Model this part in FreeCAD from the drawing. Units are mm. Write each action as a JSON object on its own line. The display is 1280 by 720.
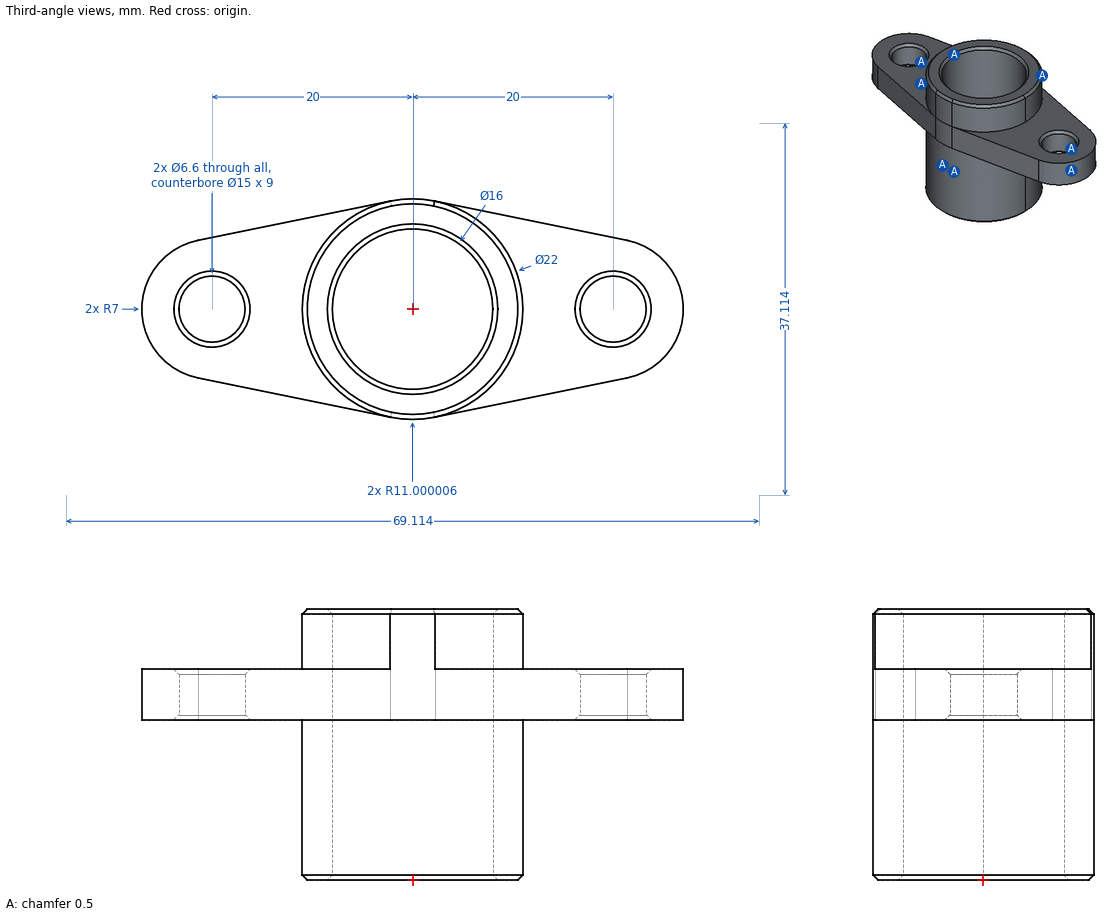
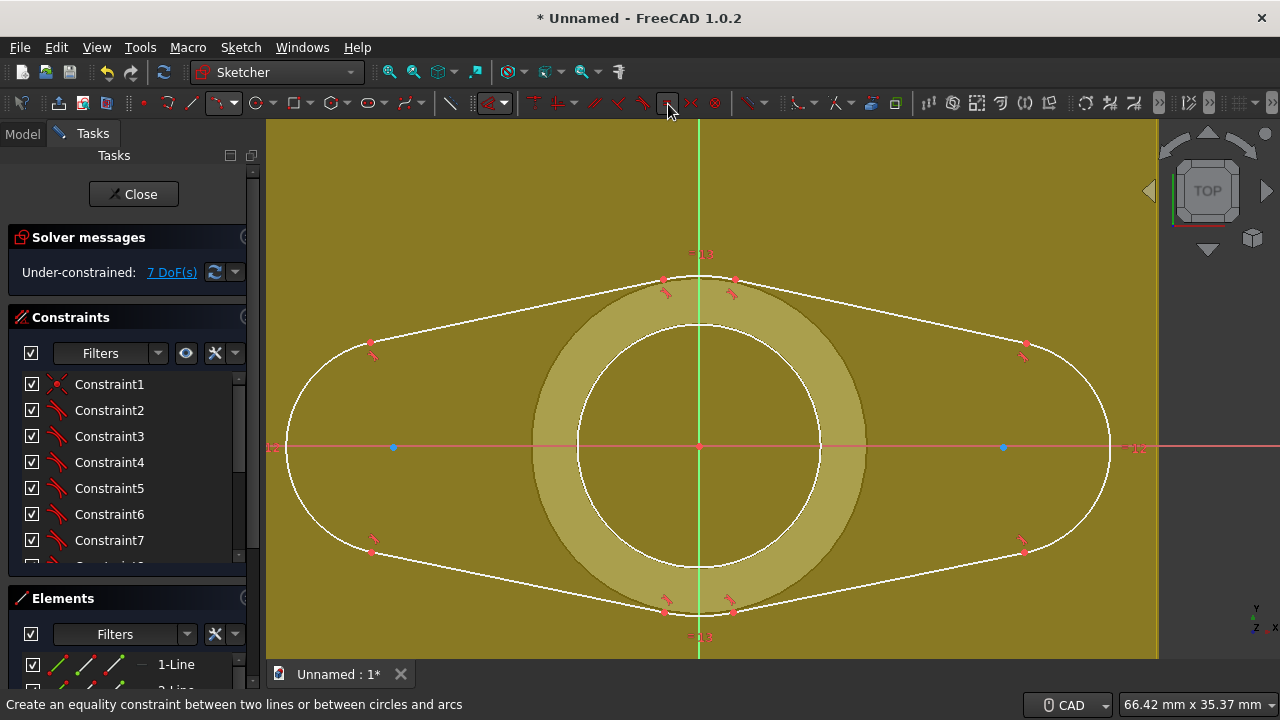
{"action": "left_click", "coordinate": [393, 447]}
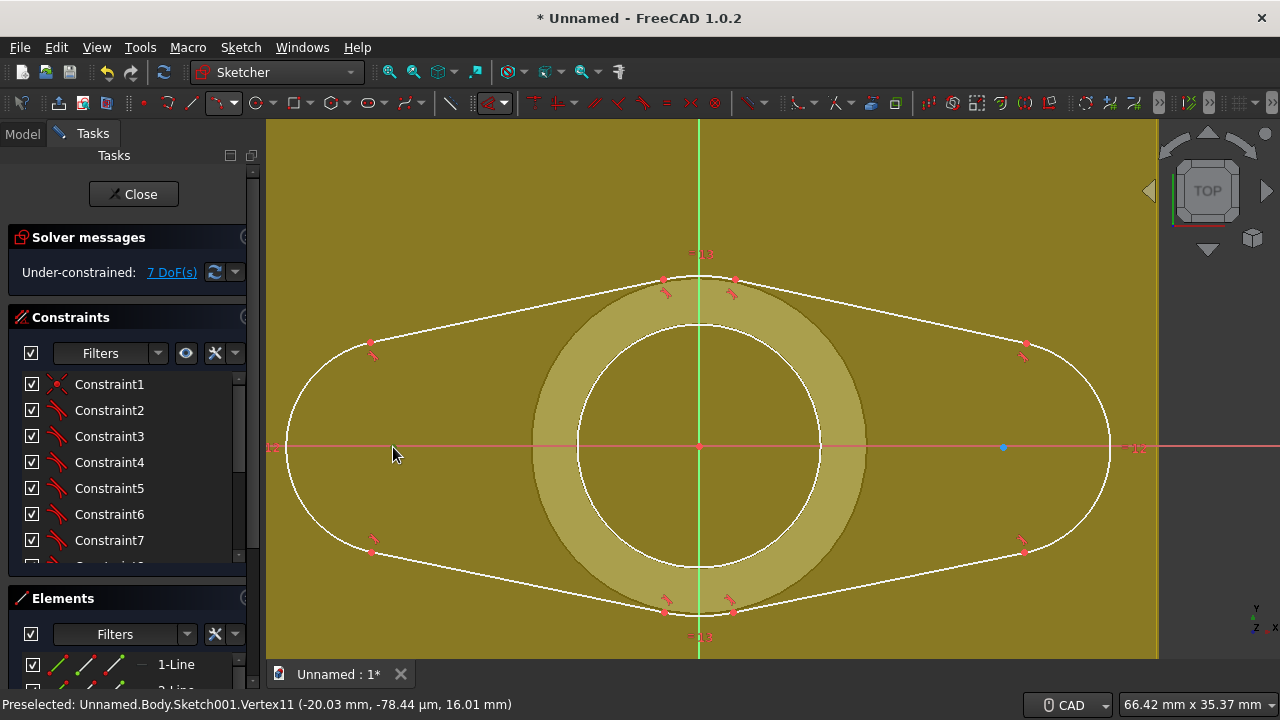
{"action": "left_click", "coordinate": [353, 446]}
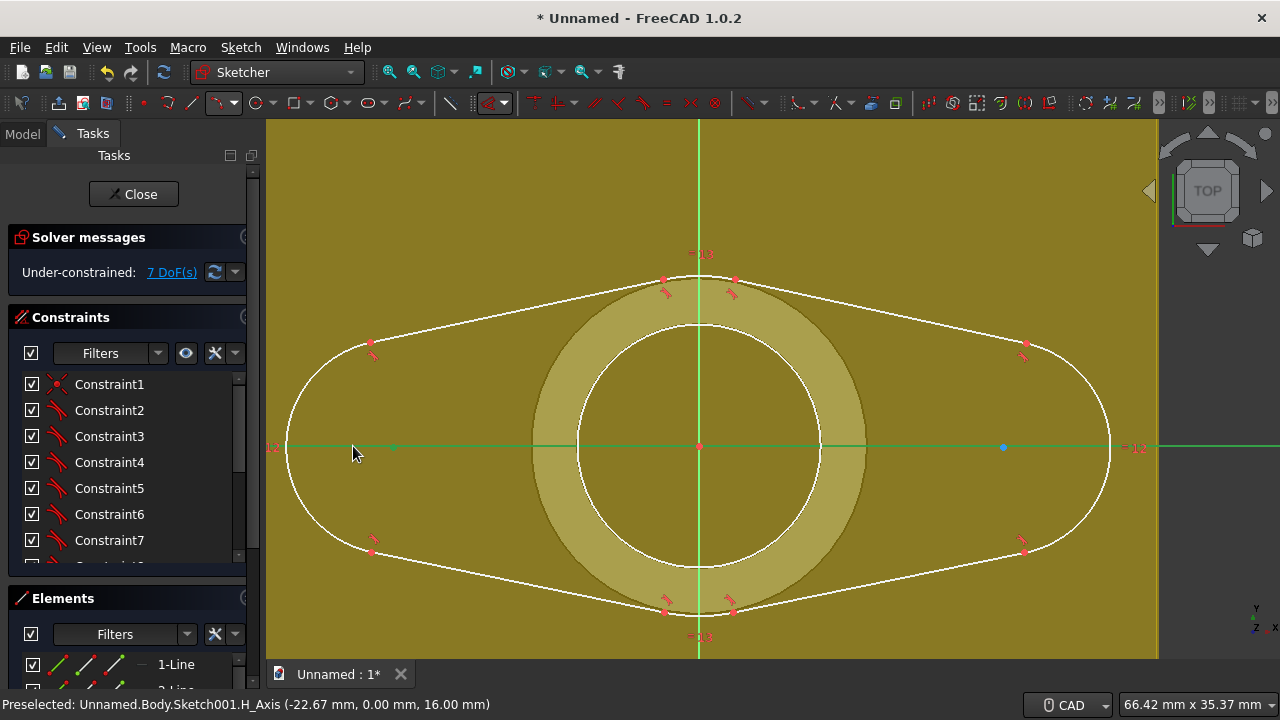
{"action": "left_click", "coordinate": [534, 104]}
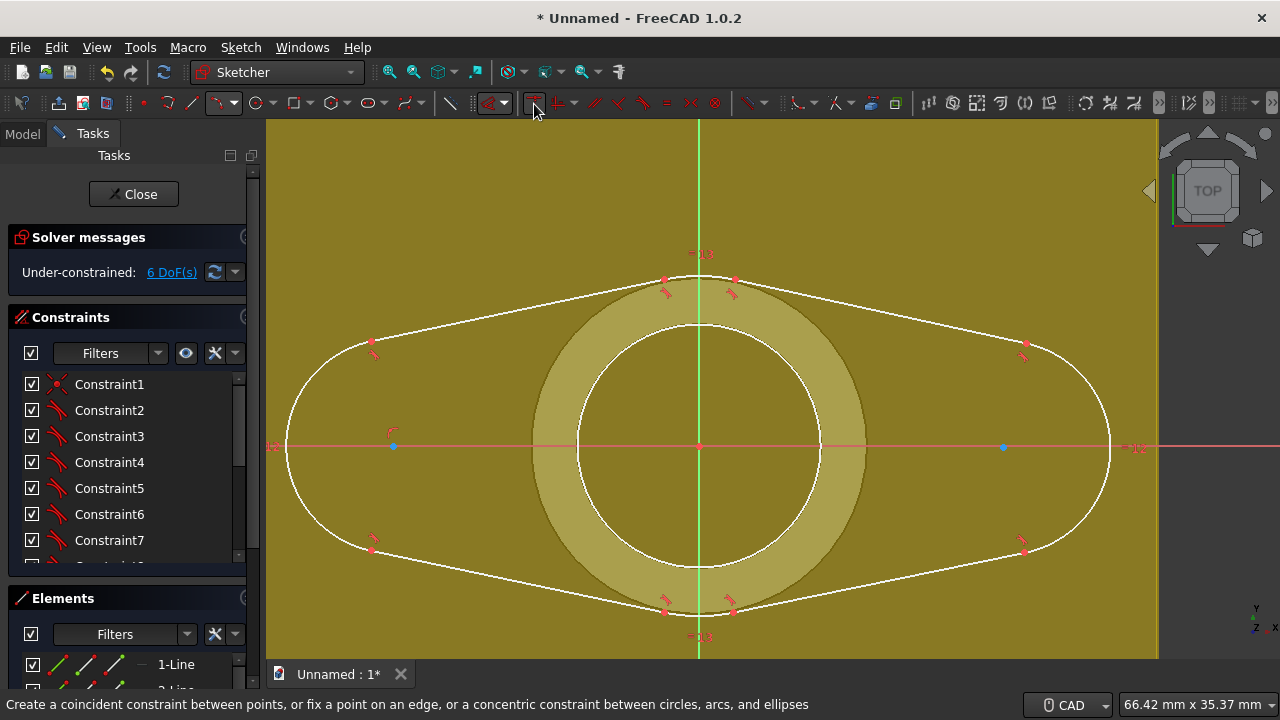
{"action": "left_click", "coordinate": [1003, 448]}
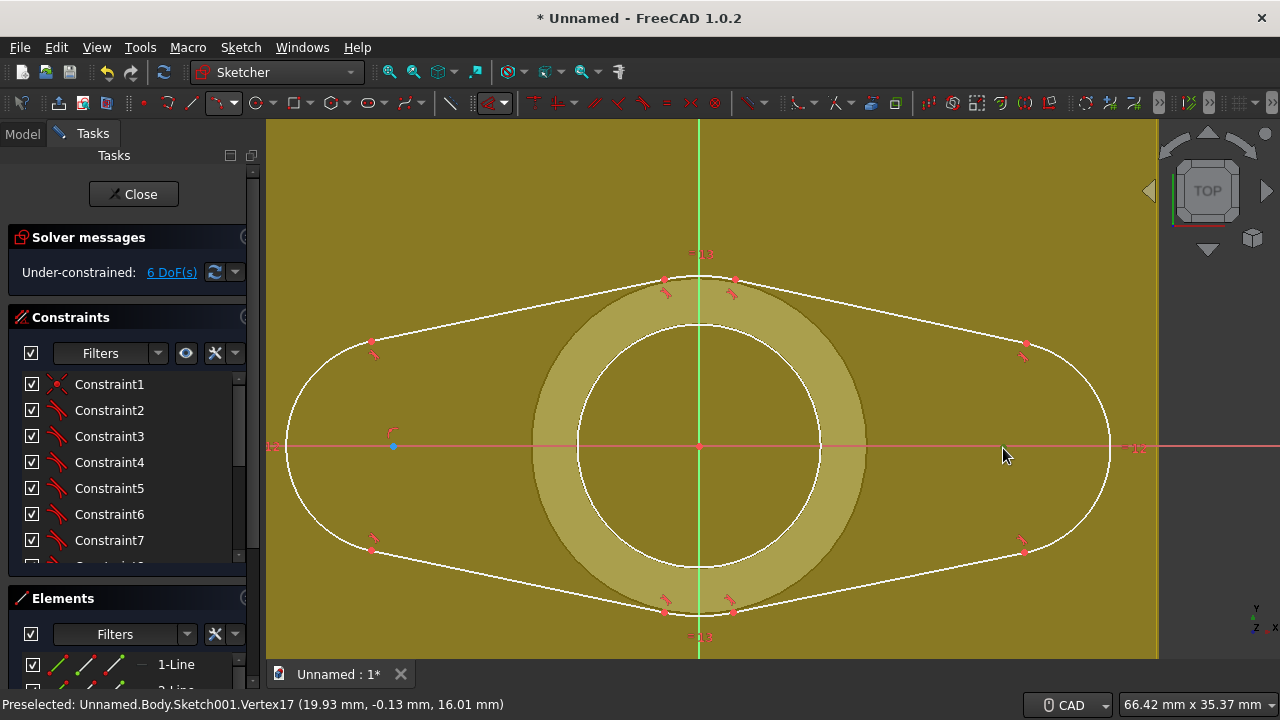
{"action": "left_click", "coordinate": [353, 446]}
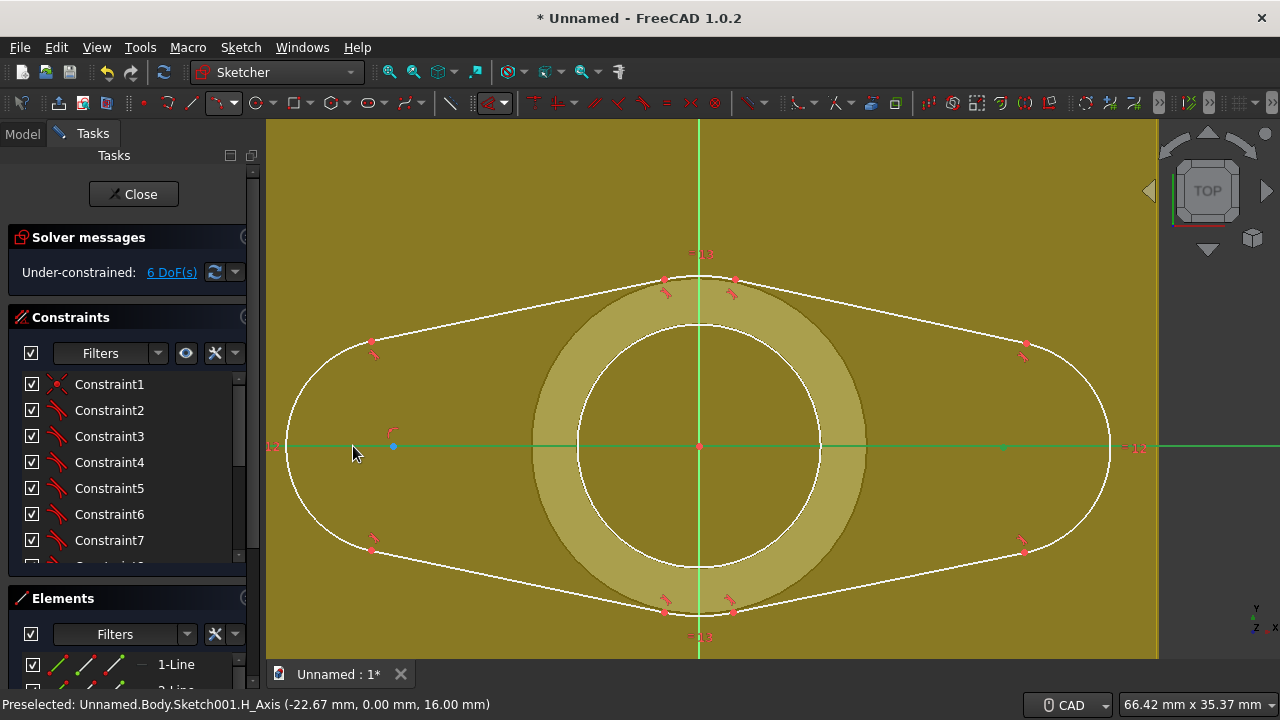
{"action": "left_click", "coordinate": [534, 104]}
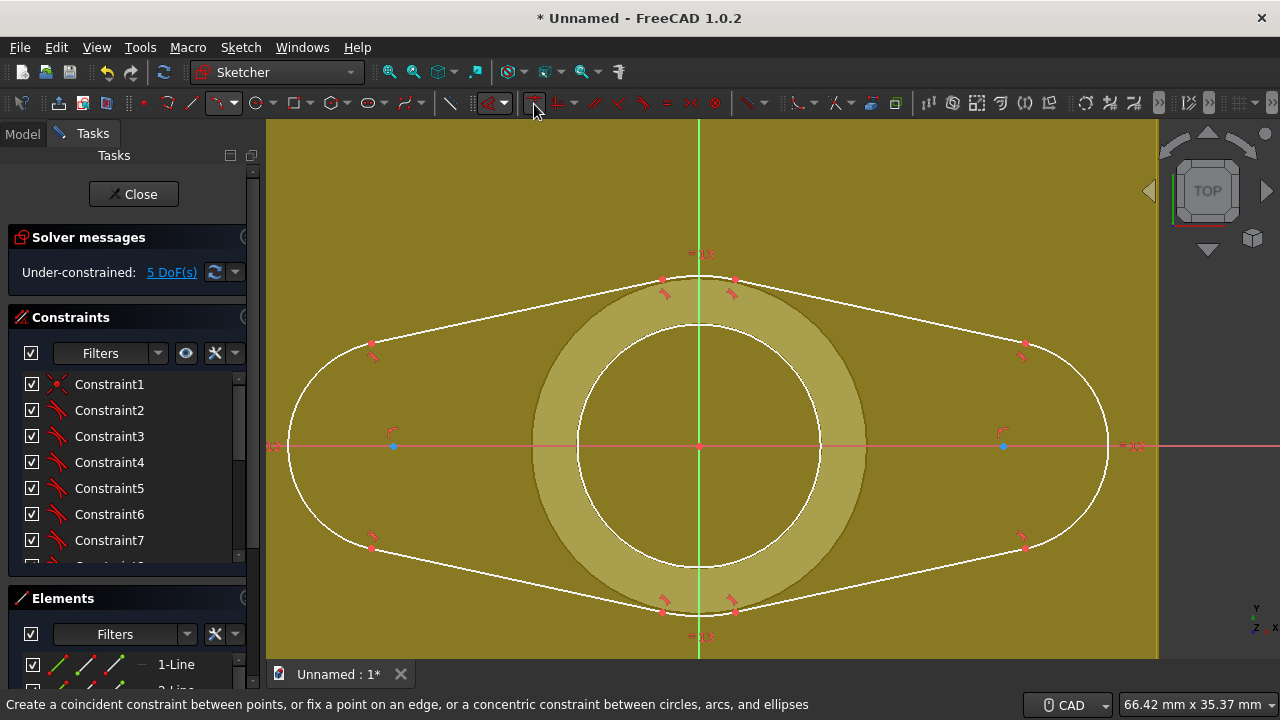
{"action": "left_click", "coordinate": [303, 392]}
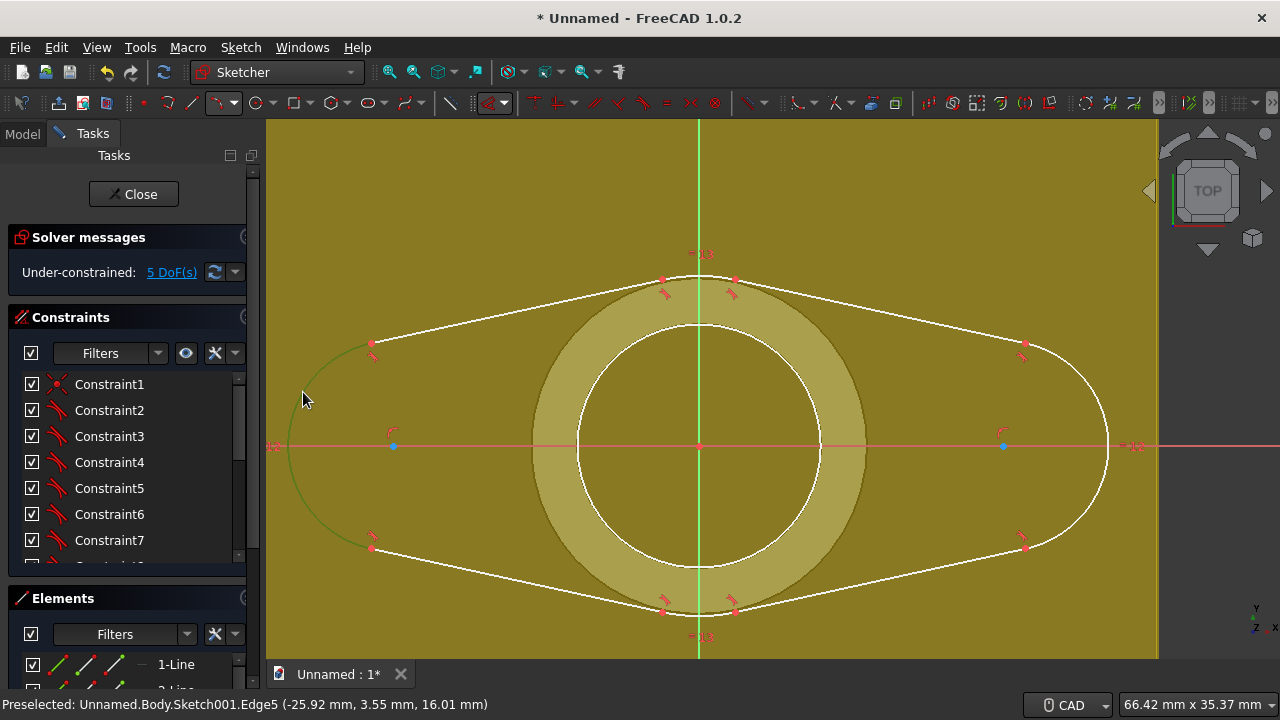
{"action": "key", "text": "k r"}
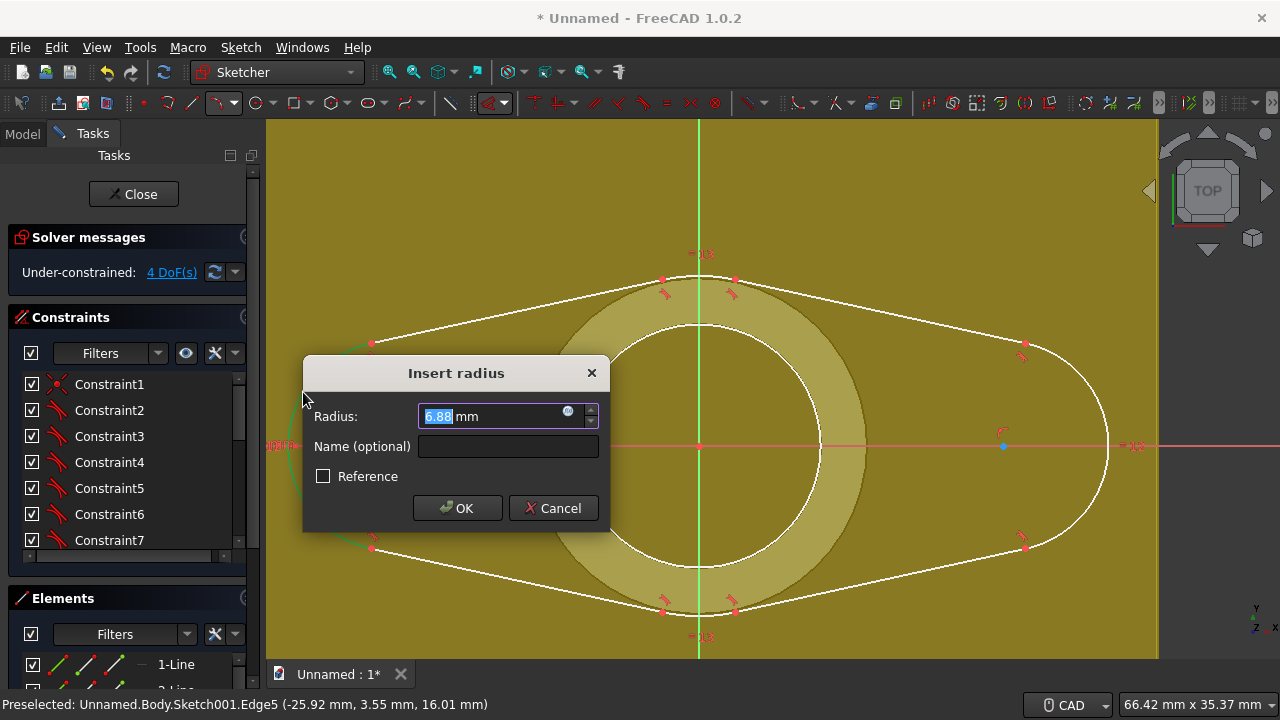
{"action": "type", "text": "7"}
{"action": "key", "text": "Return"}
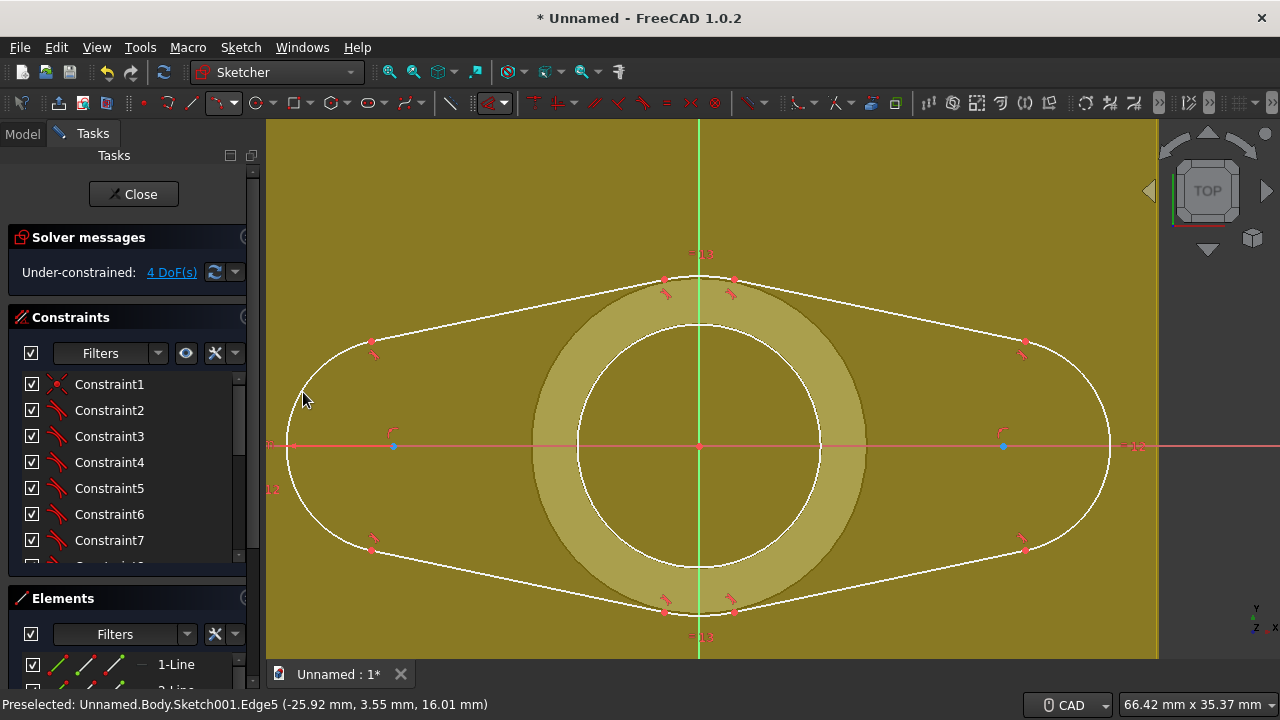
{"action": "left_click", "coordinate": [685, 615]}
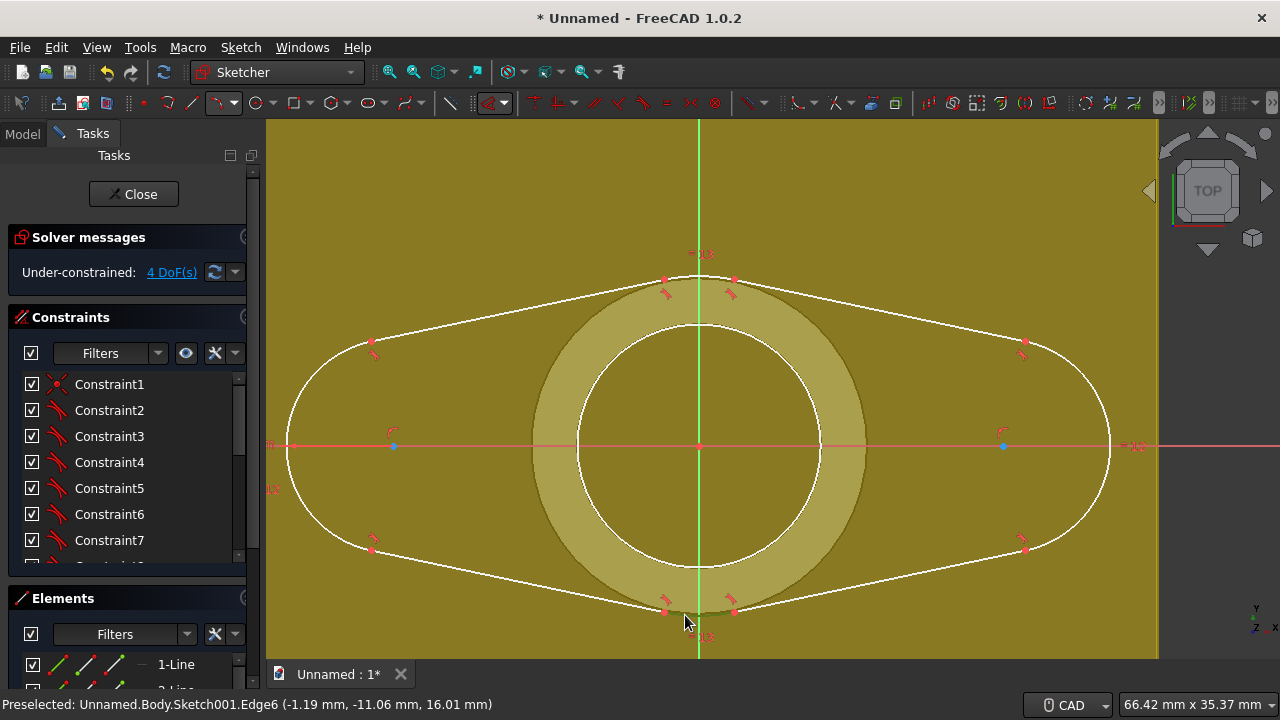
{"action": "key", "text": "k r"}